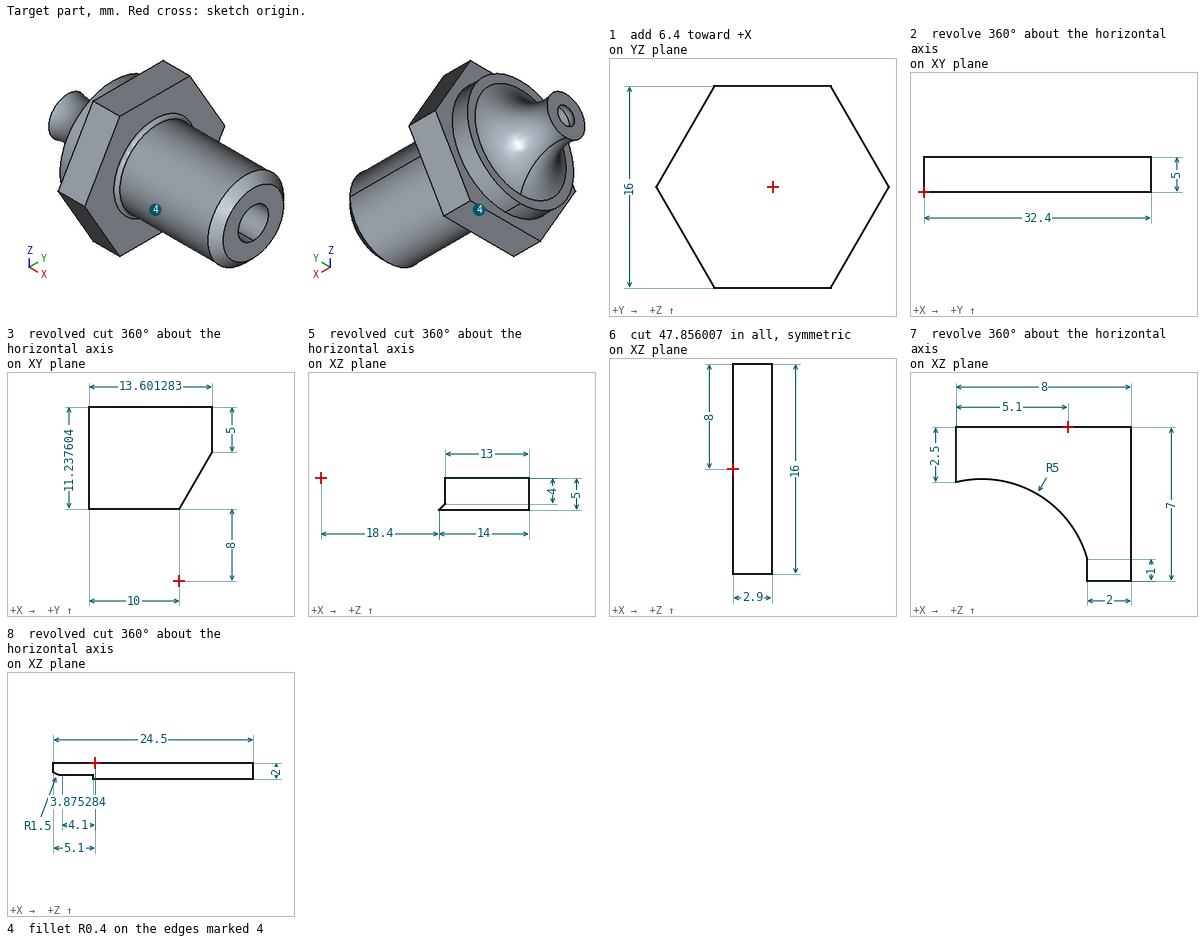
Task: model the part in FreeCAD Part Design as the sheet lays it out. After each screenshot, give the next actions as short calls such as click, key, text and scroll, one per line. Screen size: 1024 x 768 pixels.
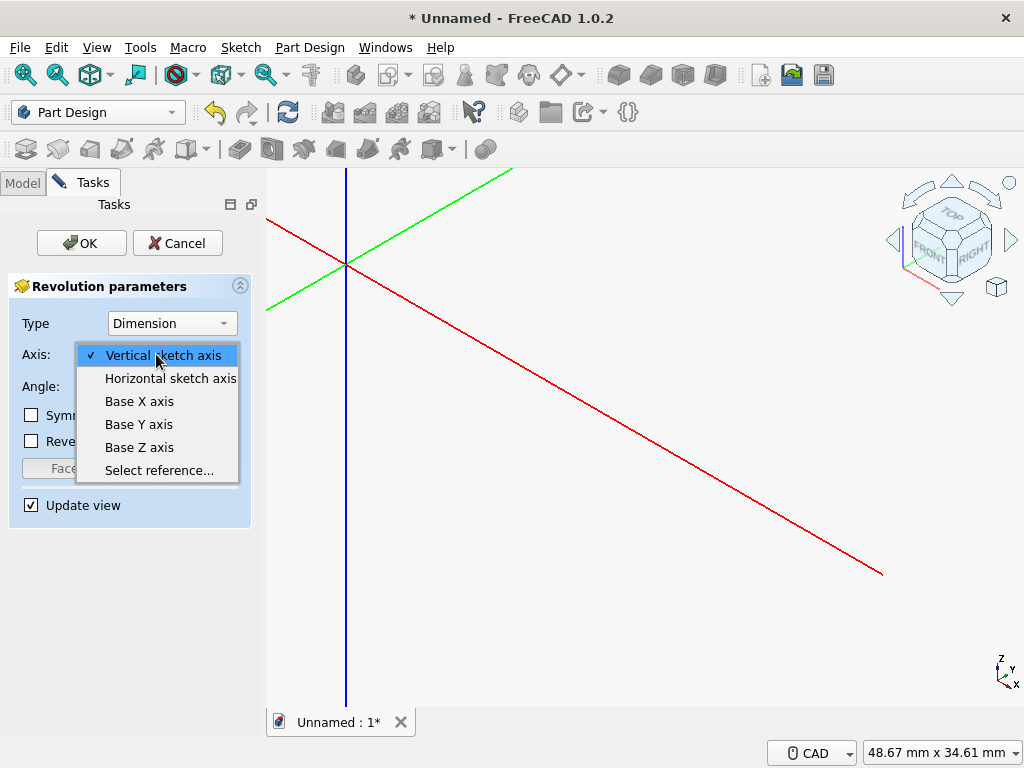
click(156, 378)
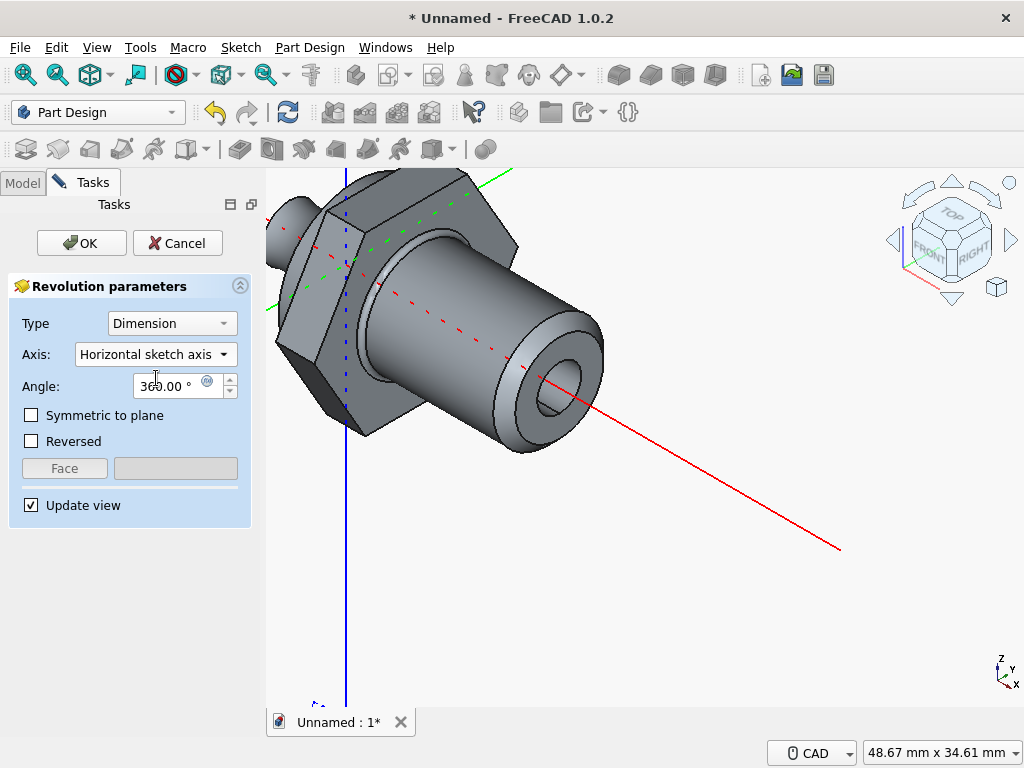
click(82, 243)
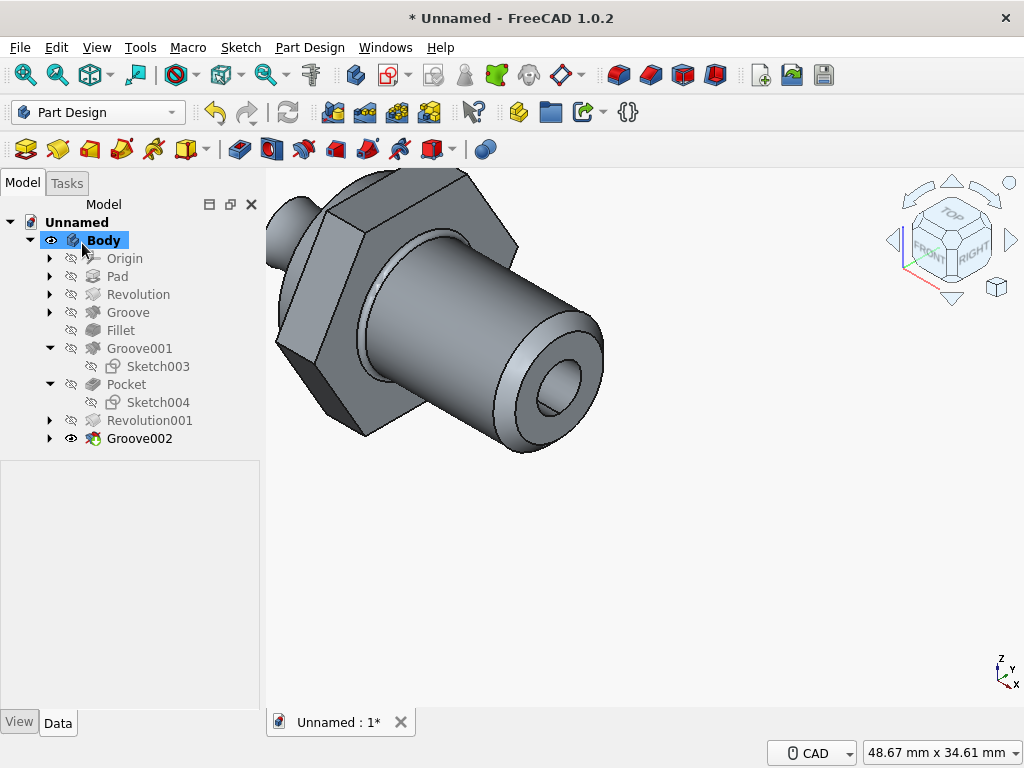
click(26, 76)